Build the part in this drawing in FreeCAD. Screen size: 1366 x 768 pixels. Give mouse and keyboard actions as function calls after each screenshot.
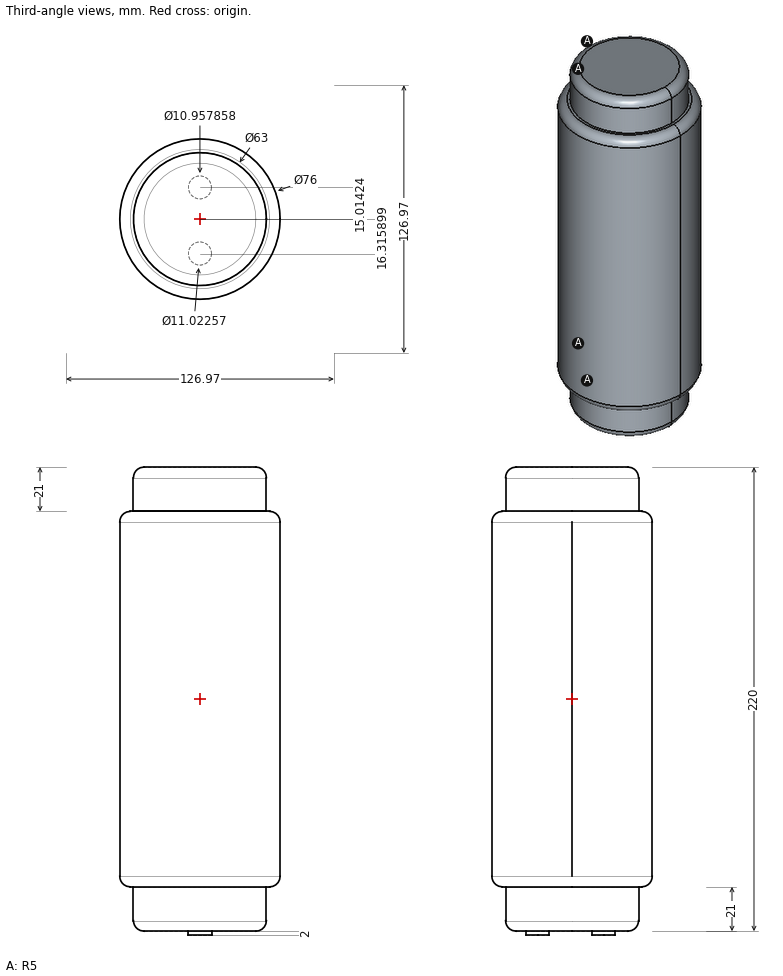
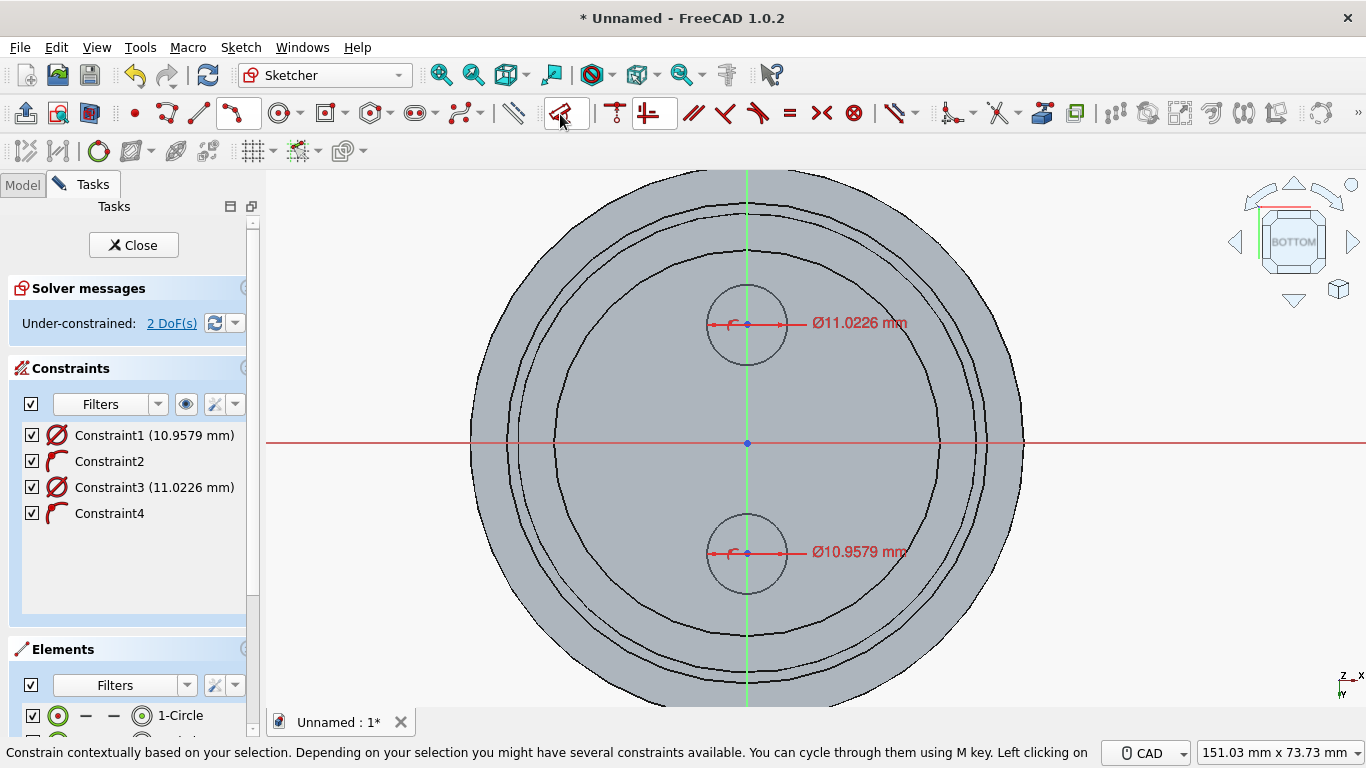
click(747, 554)
click(781, 499)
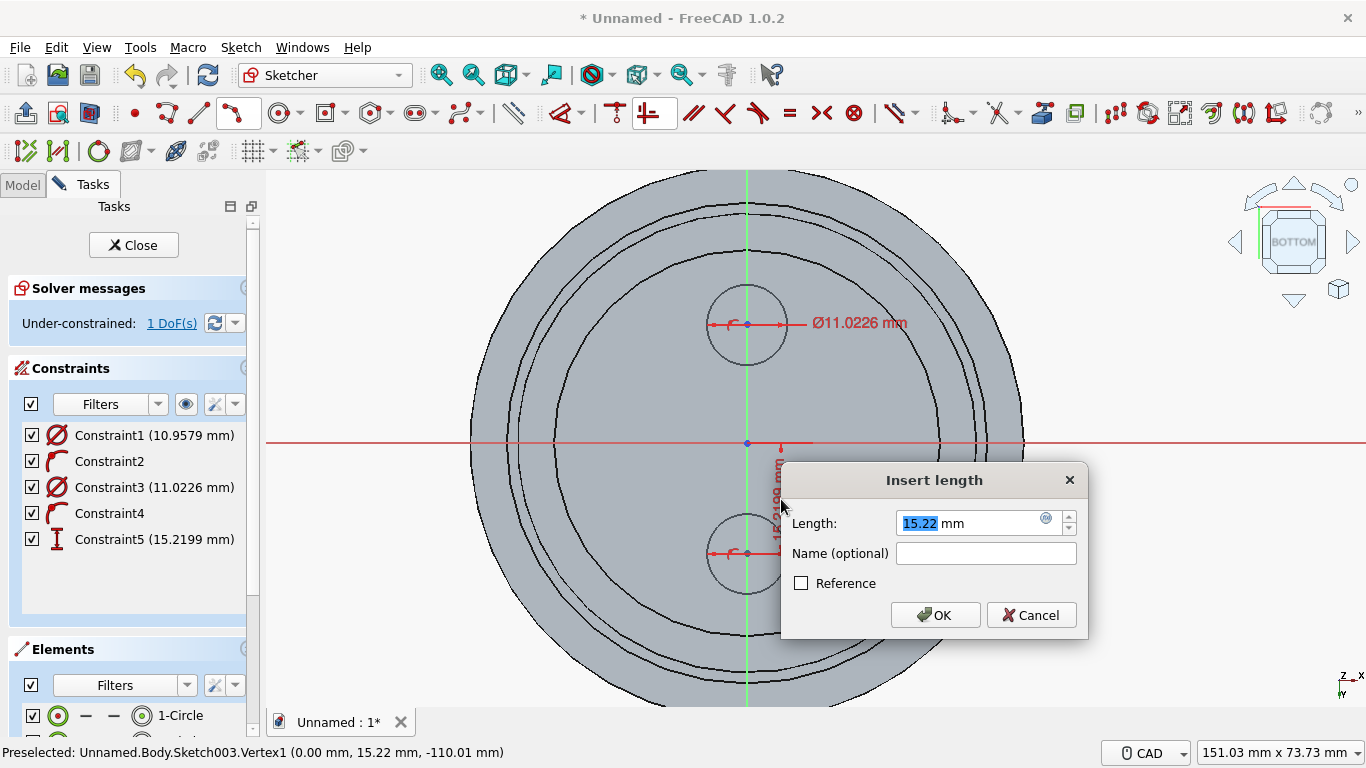
text(15.01424)
key(Return)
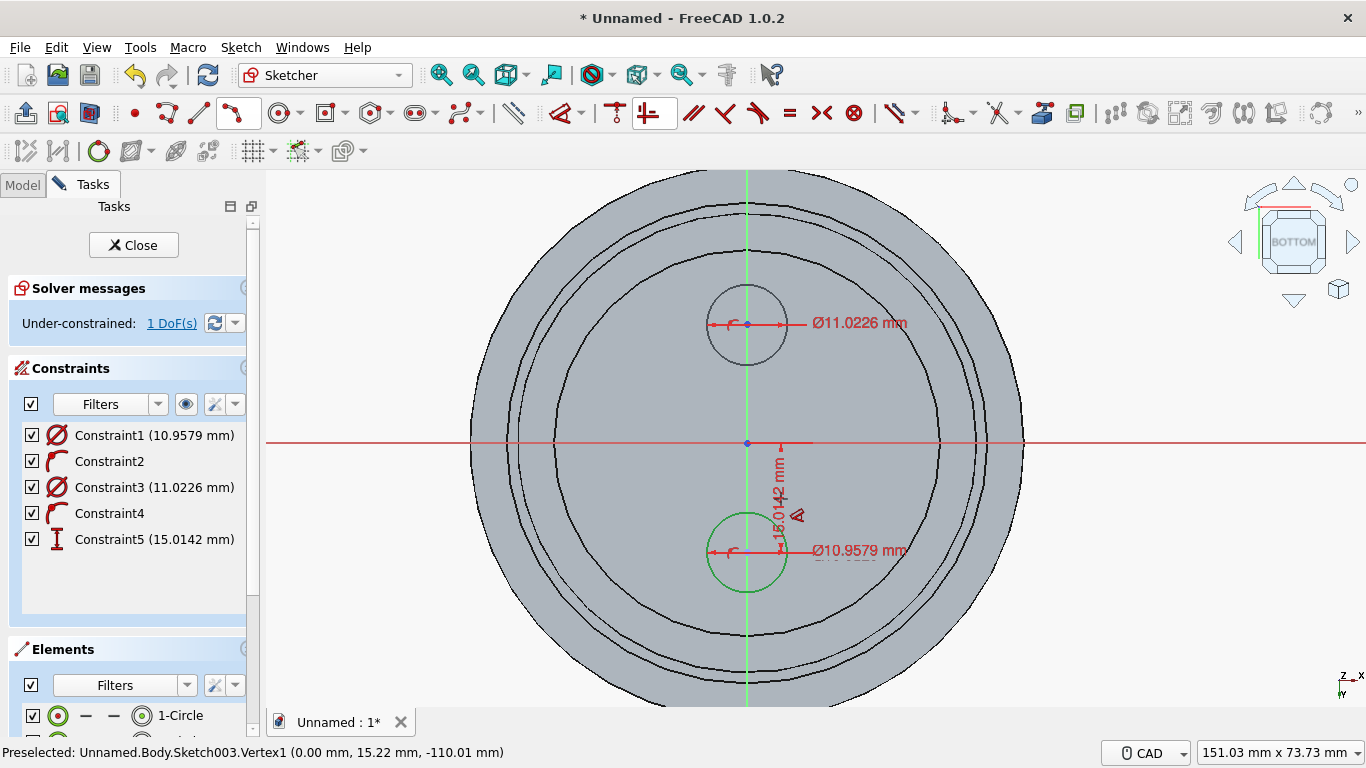
click(747, 325)
click(781, 384)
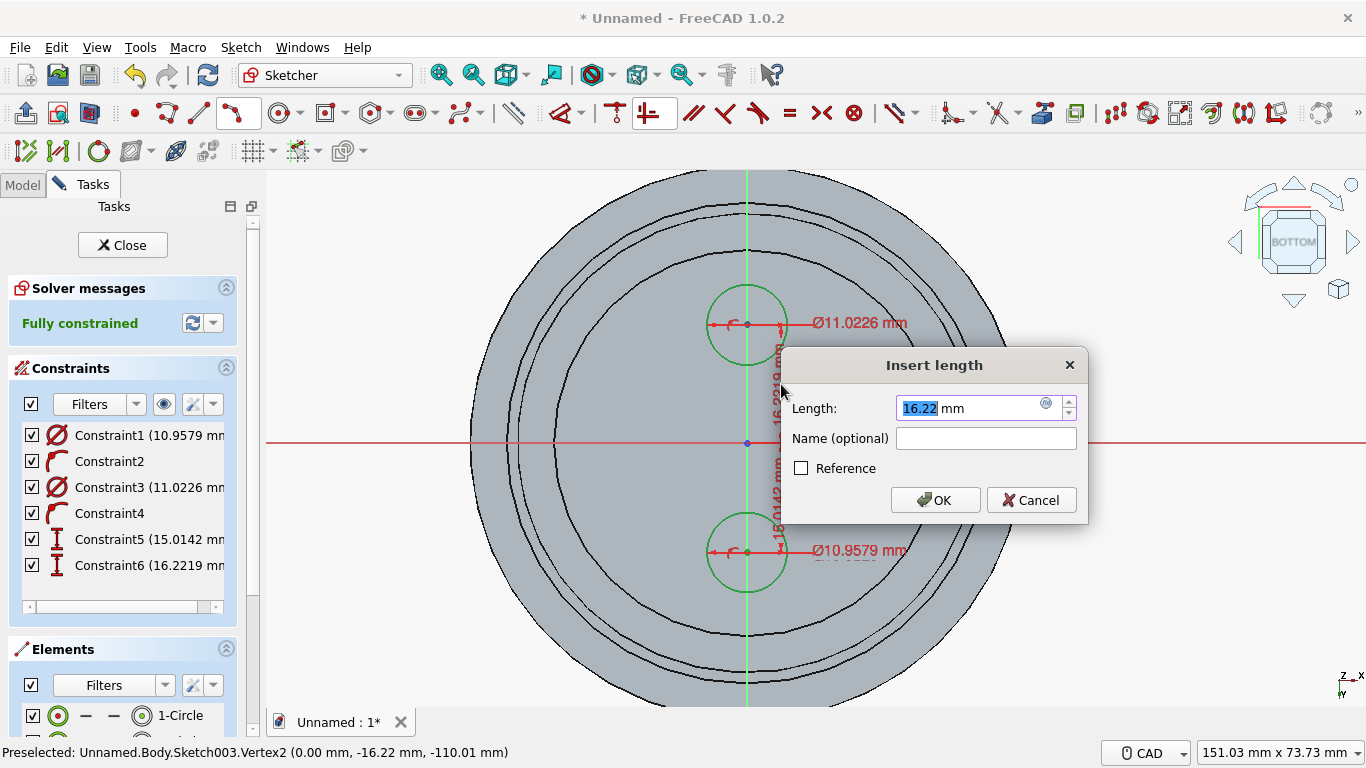
text(16.315899)
key(Return)
key(Escape)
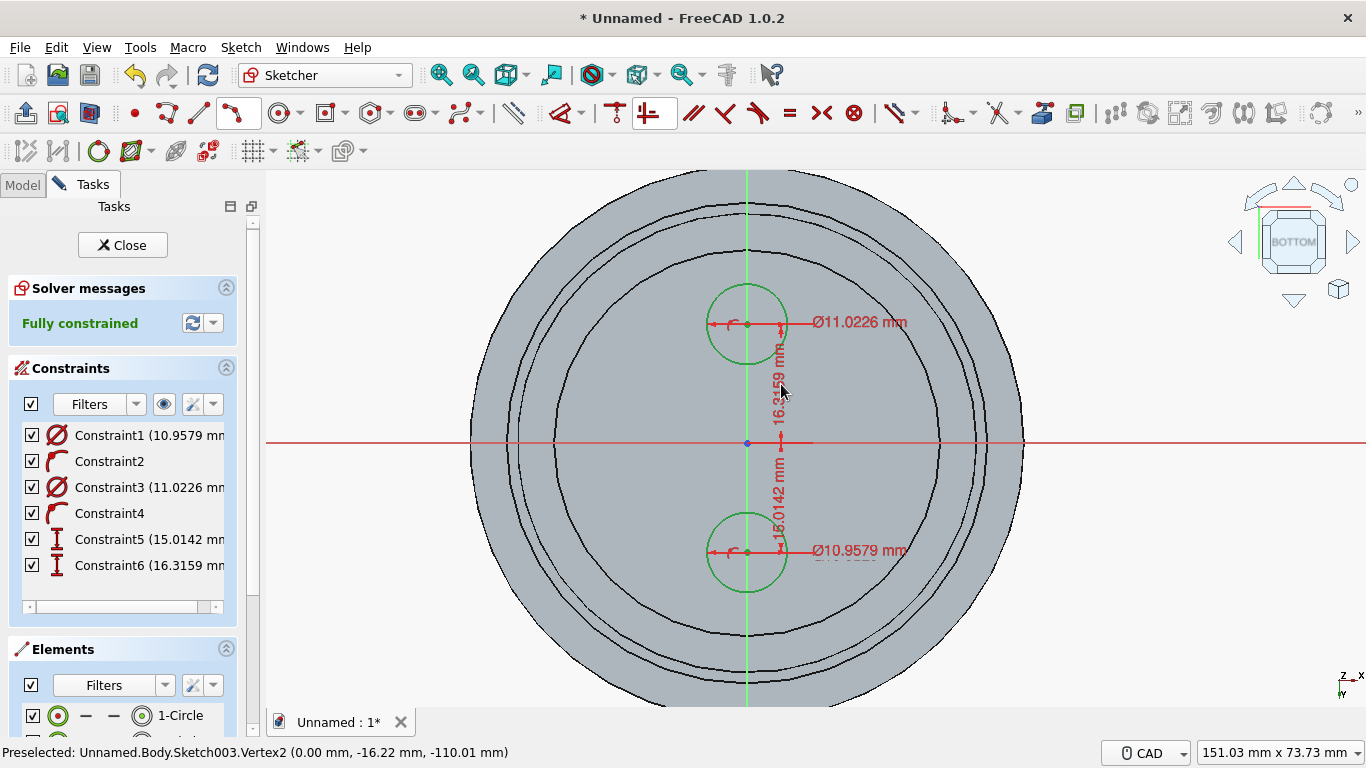
click(123, 245)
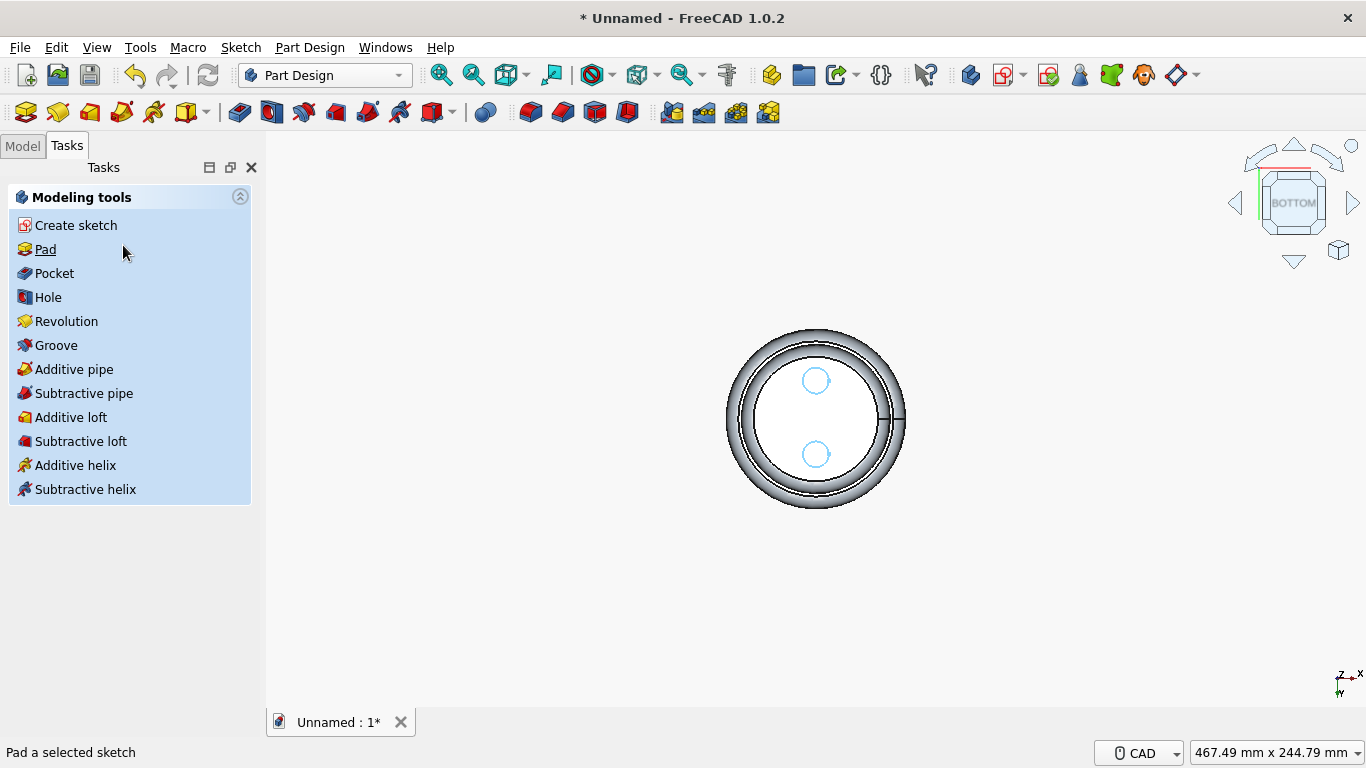
click(26, 112)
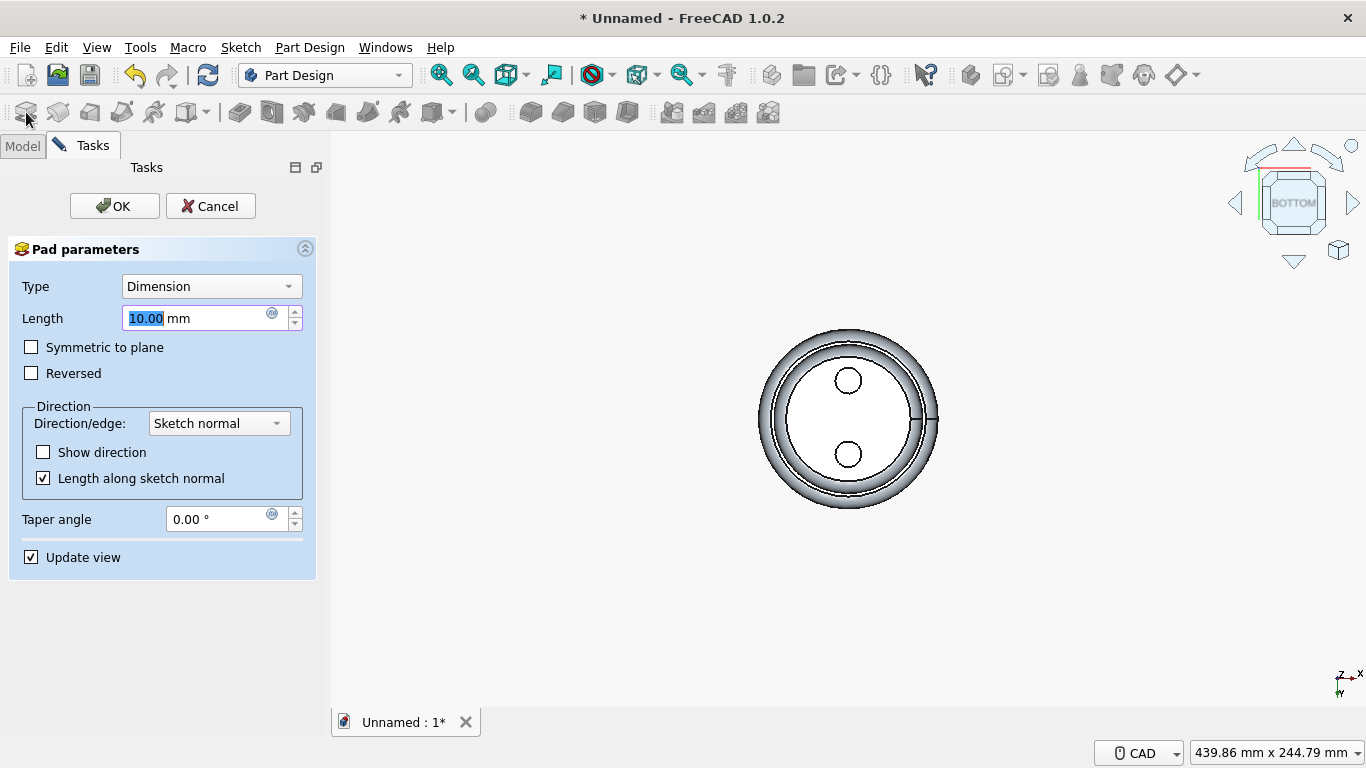
text(2)
key(Tab)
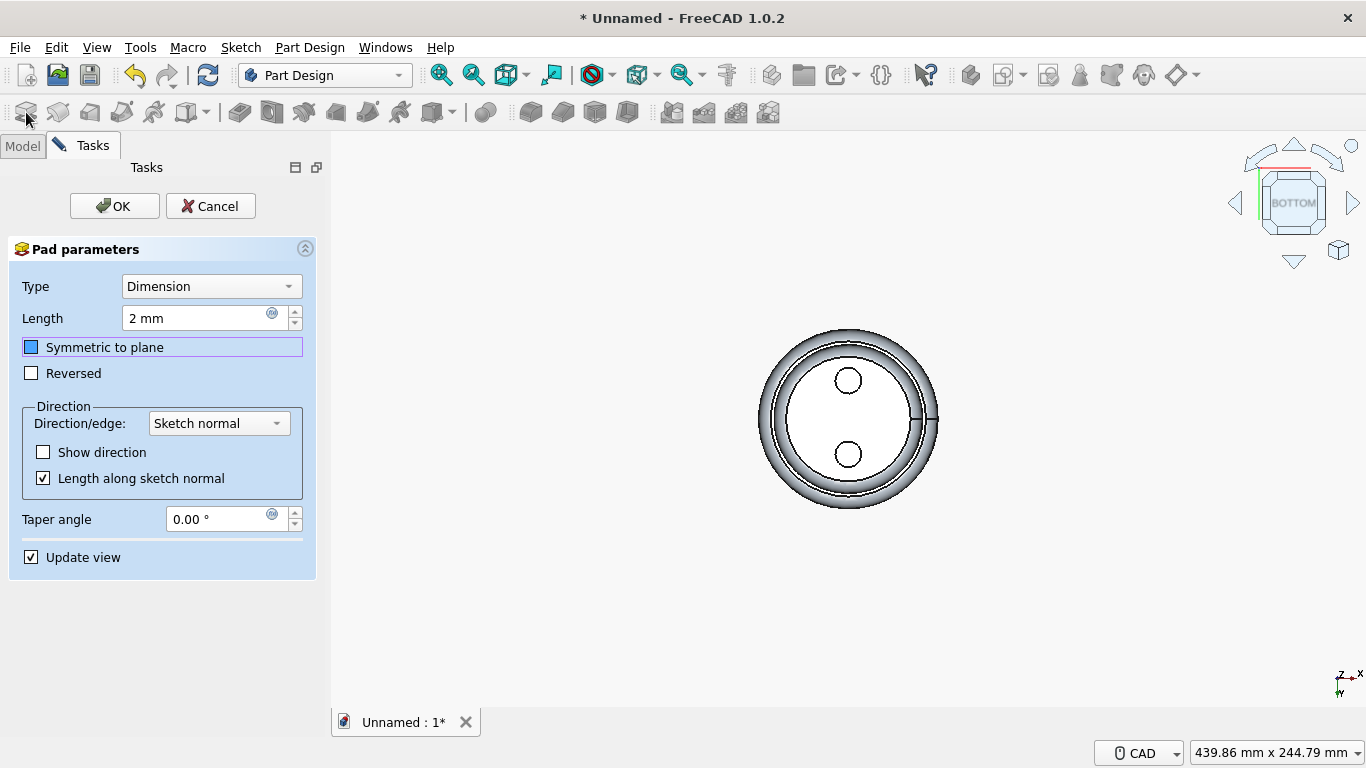
click(115, 206)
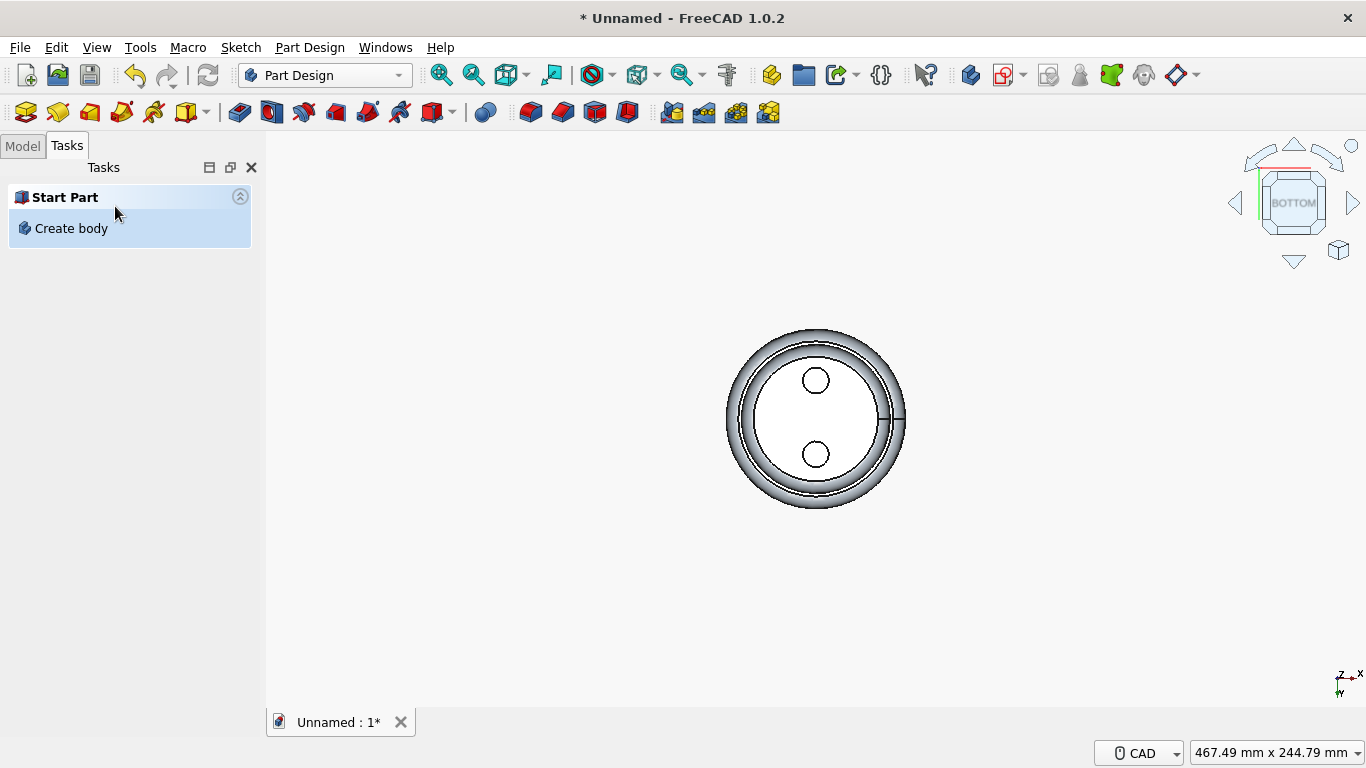
key(0)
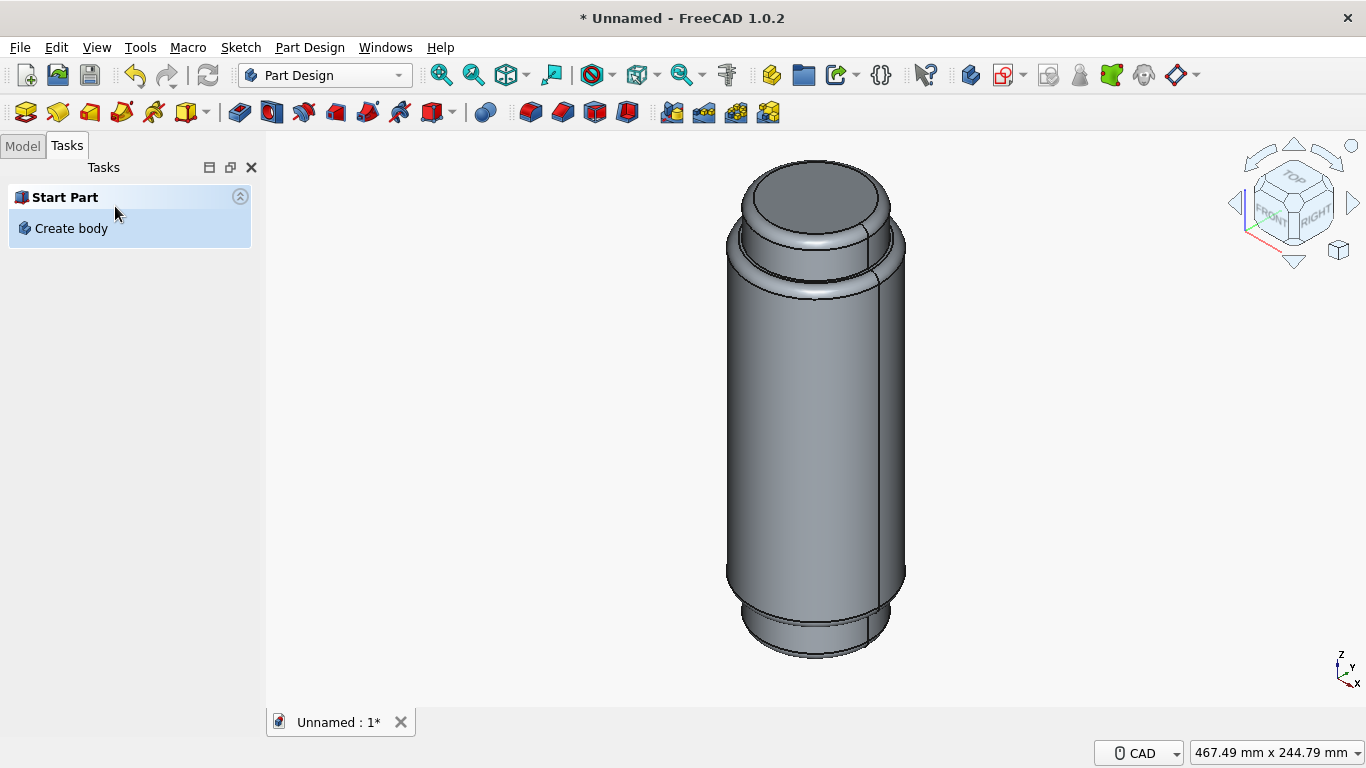
click(442, 76)